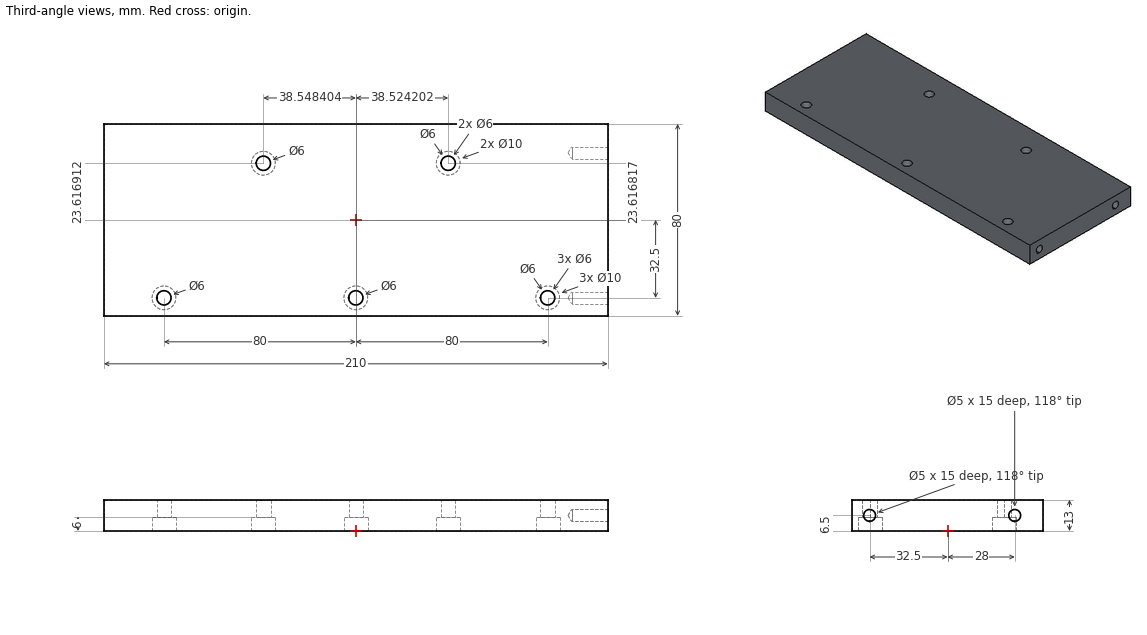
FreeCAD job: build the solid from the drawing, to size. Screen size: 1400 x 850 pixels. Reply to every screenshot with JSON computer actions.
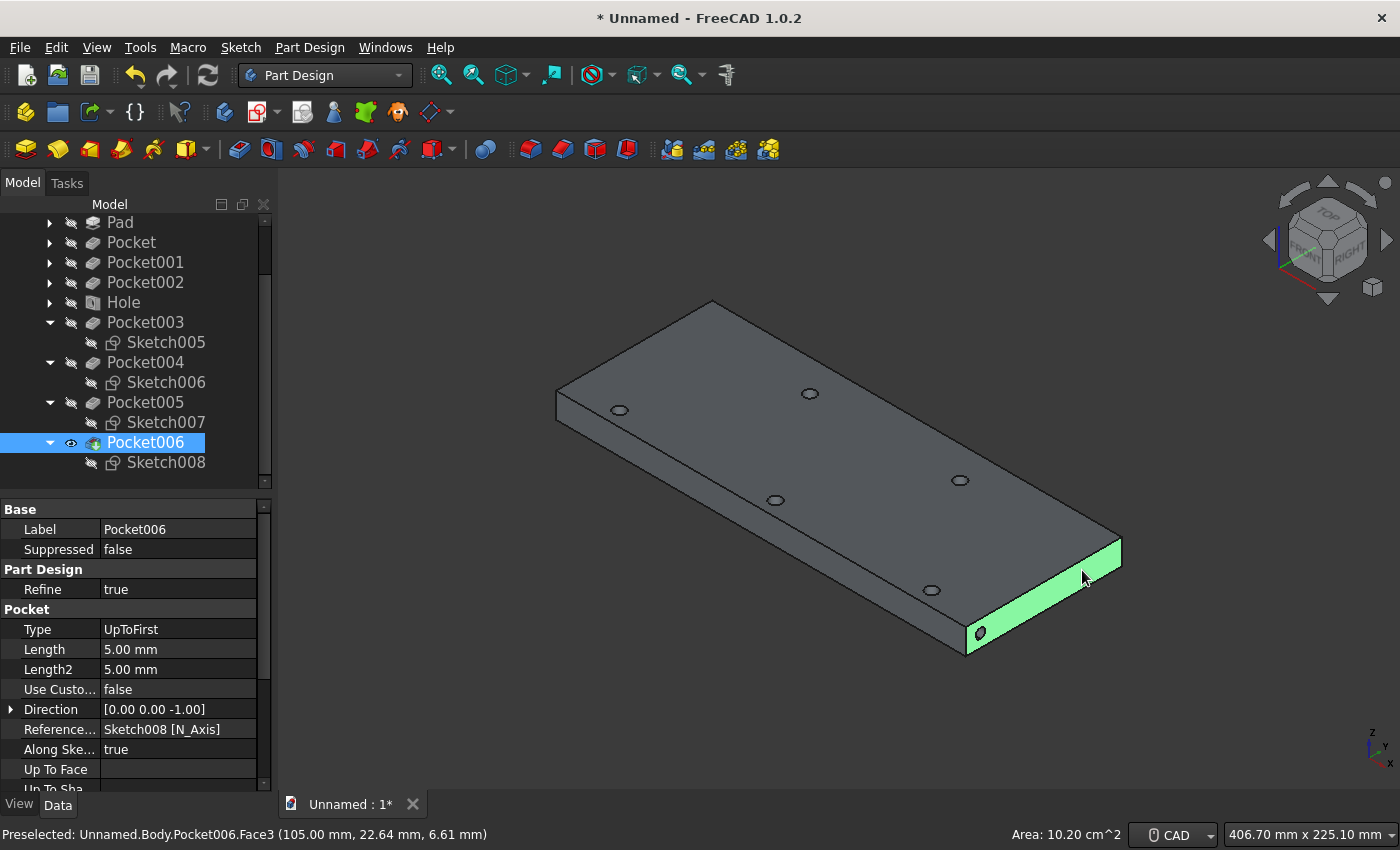
{"action": "left_click", "coordinate": [258, 112]}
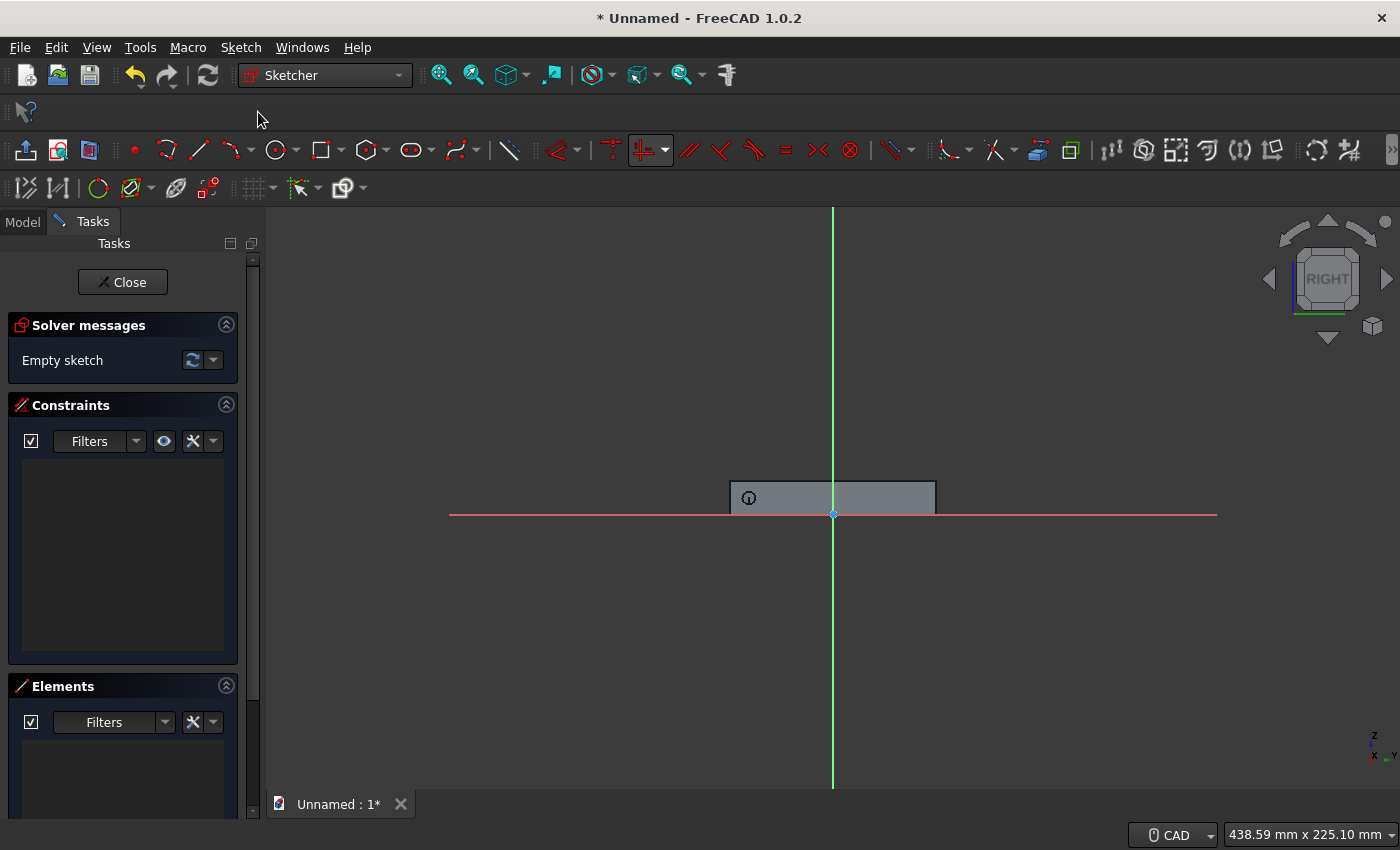
{"action": "scroll", "coordinate": [913, 498], "scroll_direction": "up", "scroll_amount": 15}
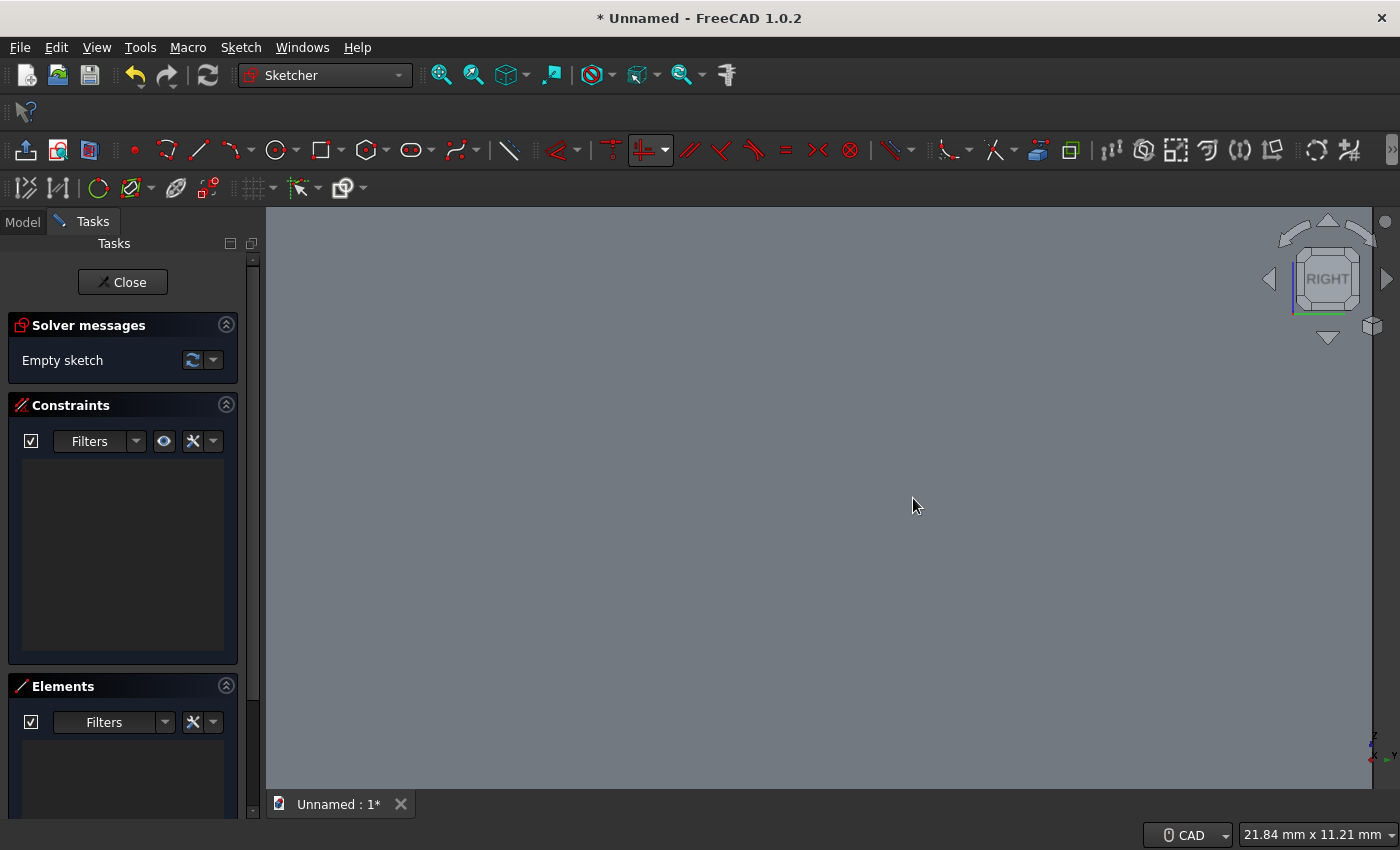
{"action": "scroll", "coordinate": [719, 469], "scroll_direction": "up", "scroll_amount": 2}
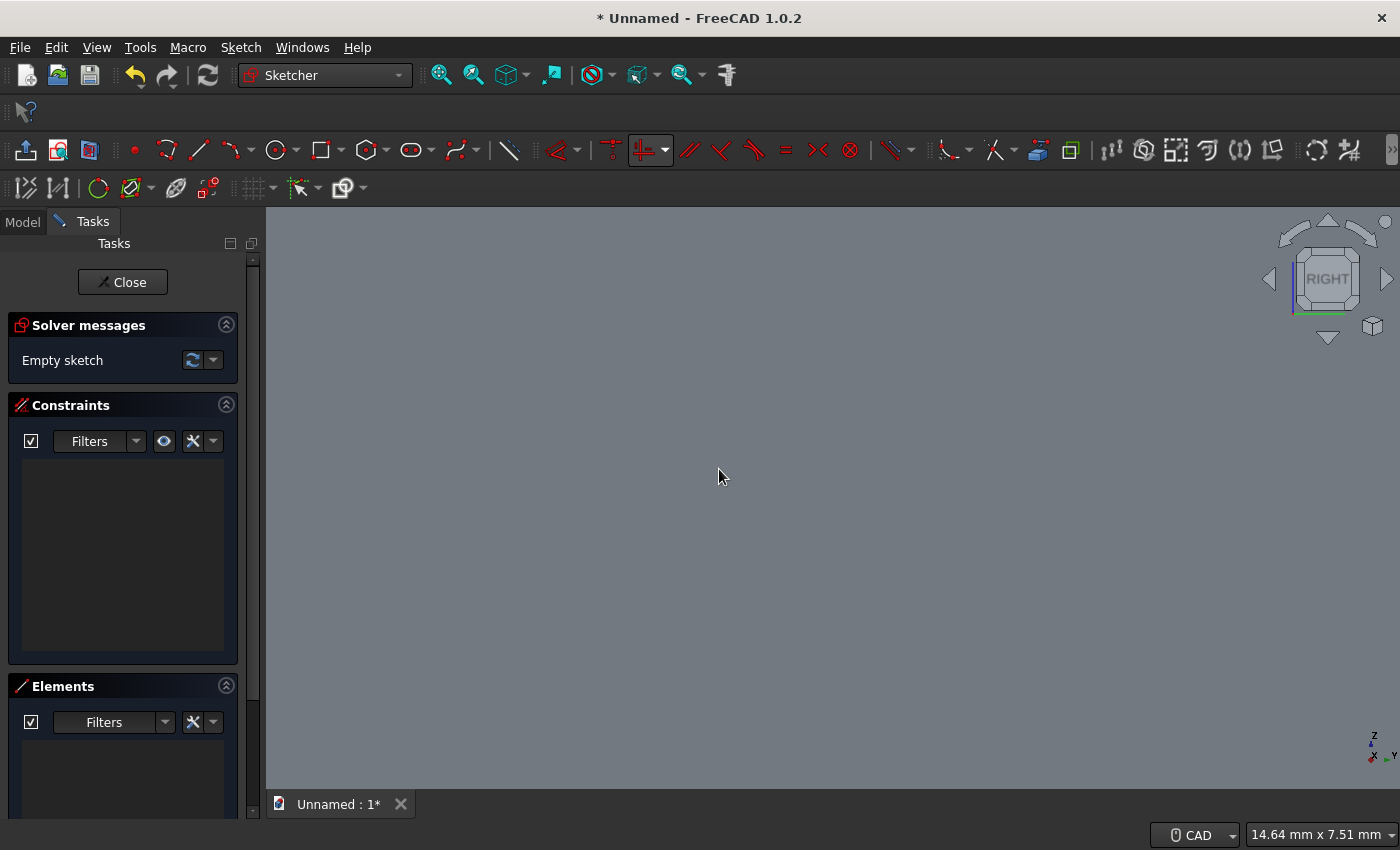
{"action": "key", "text": "g c"}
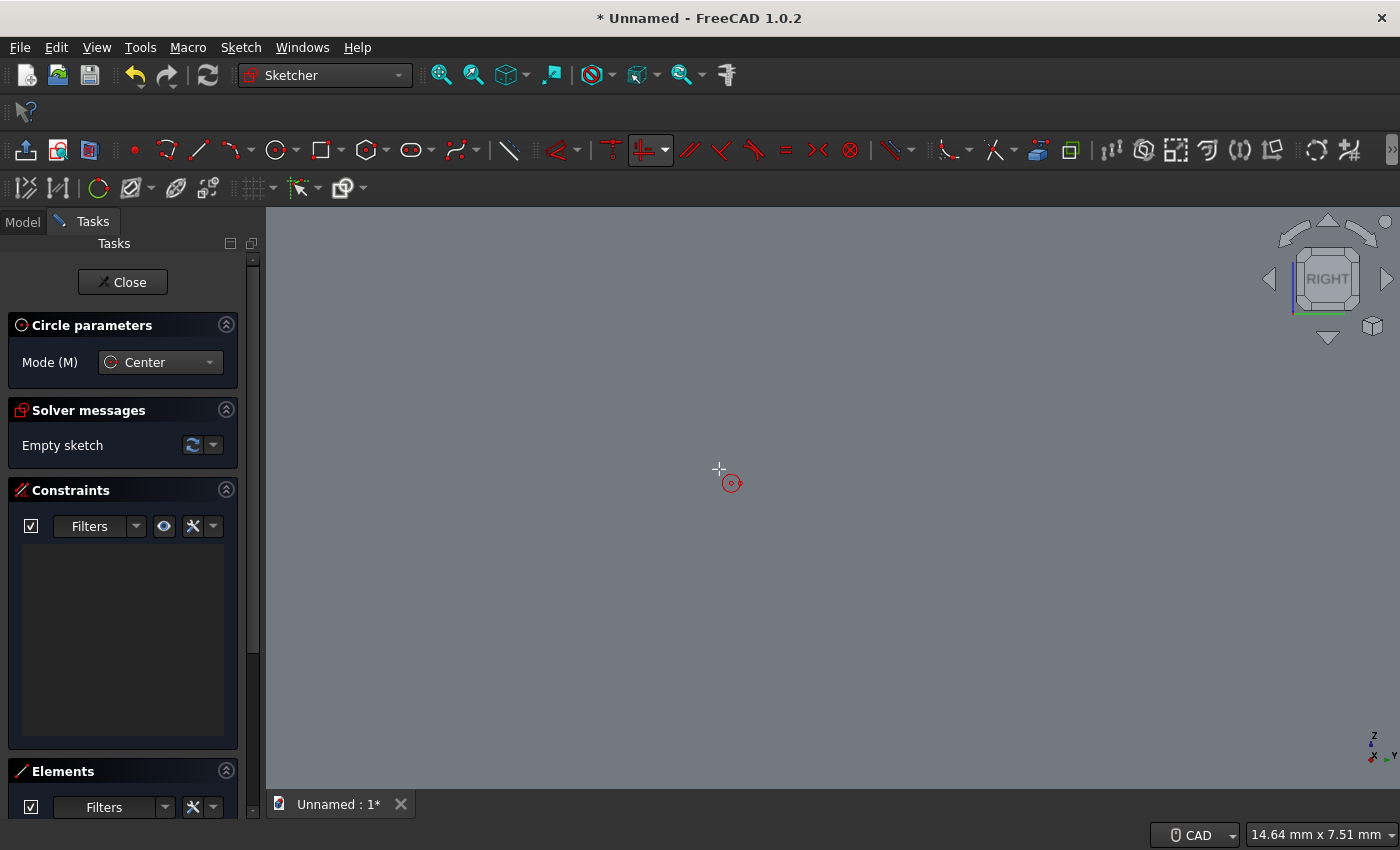
{"action": "left_click", "coordinate": [764, 498]}
{"action": "left_click", "coordinate": [901, 361]}
{"action": "key", "text": "Escape"}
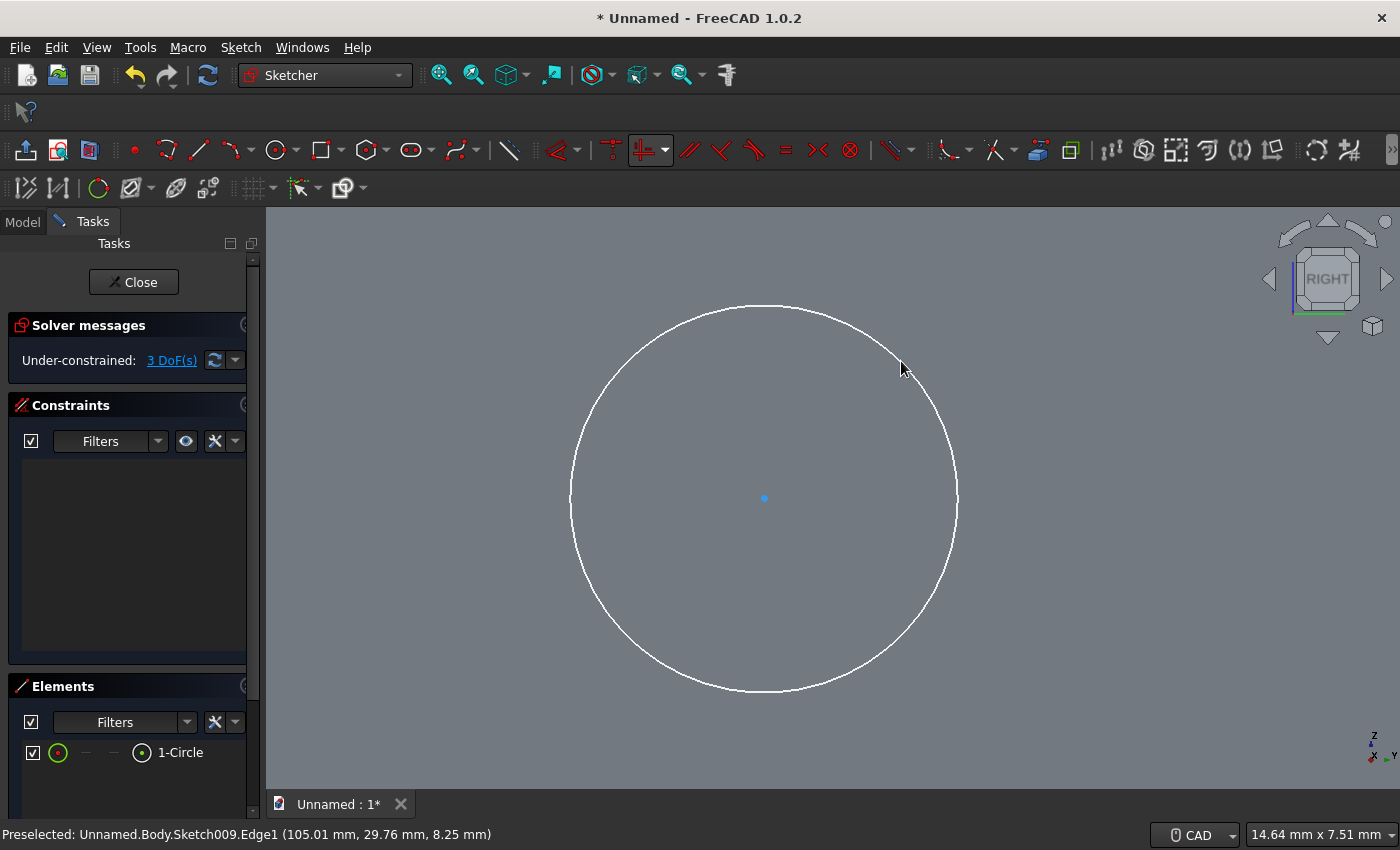
{"action": "left_click", "coordinate": [556, 150]}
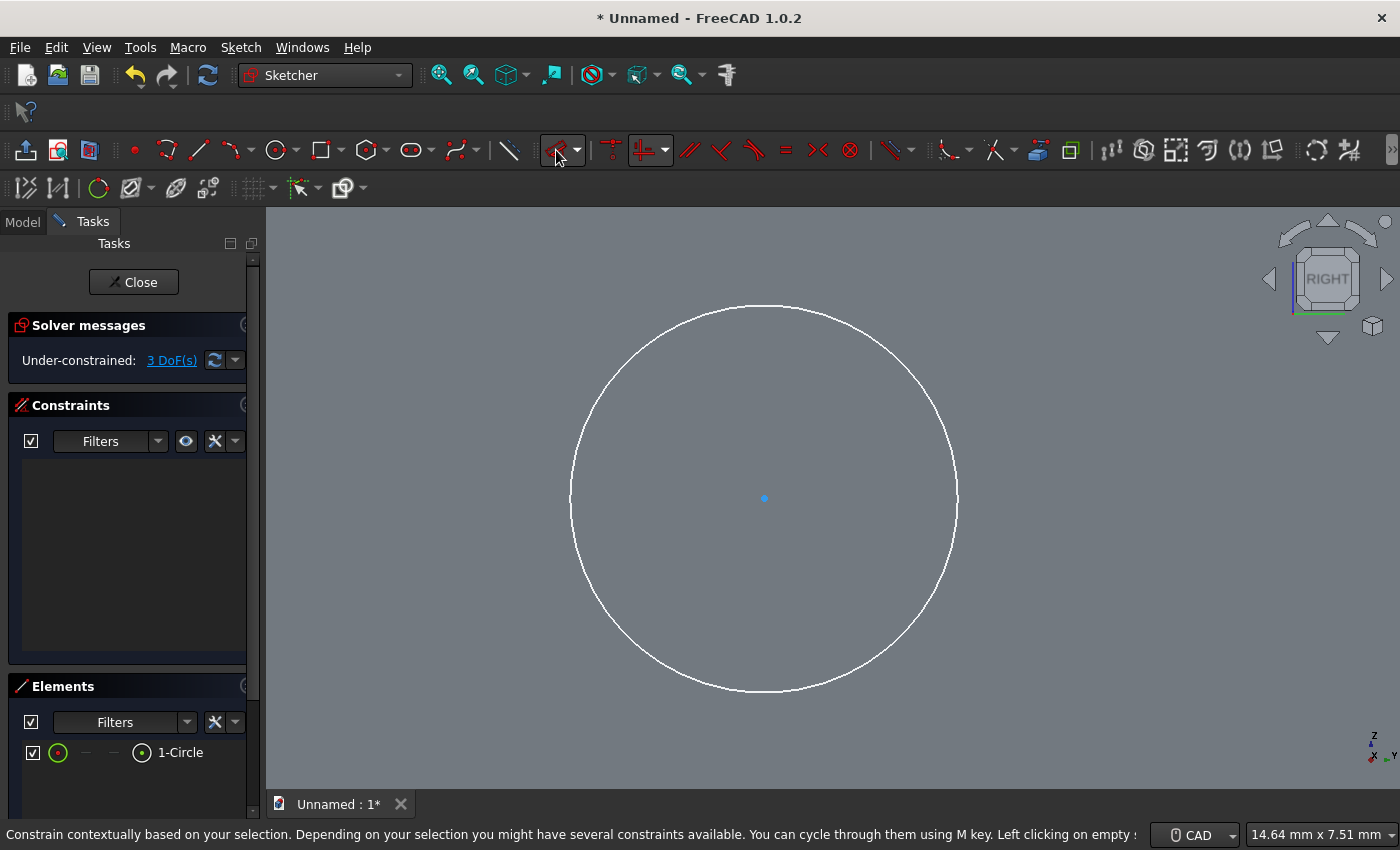
{"action": "left_click", "coordinate": [901, 362]}
{"action": "left_click", "coordinate": [924, 339]}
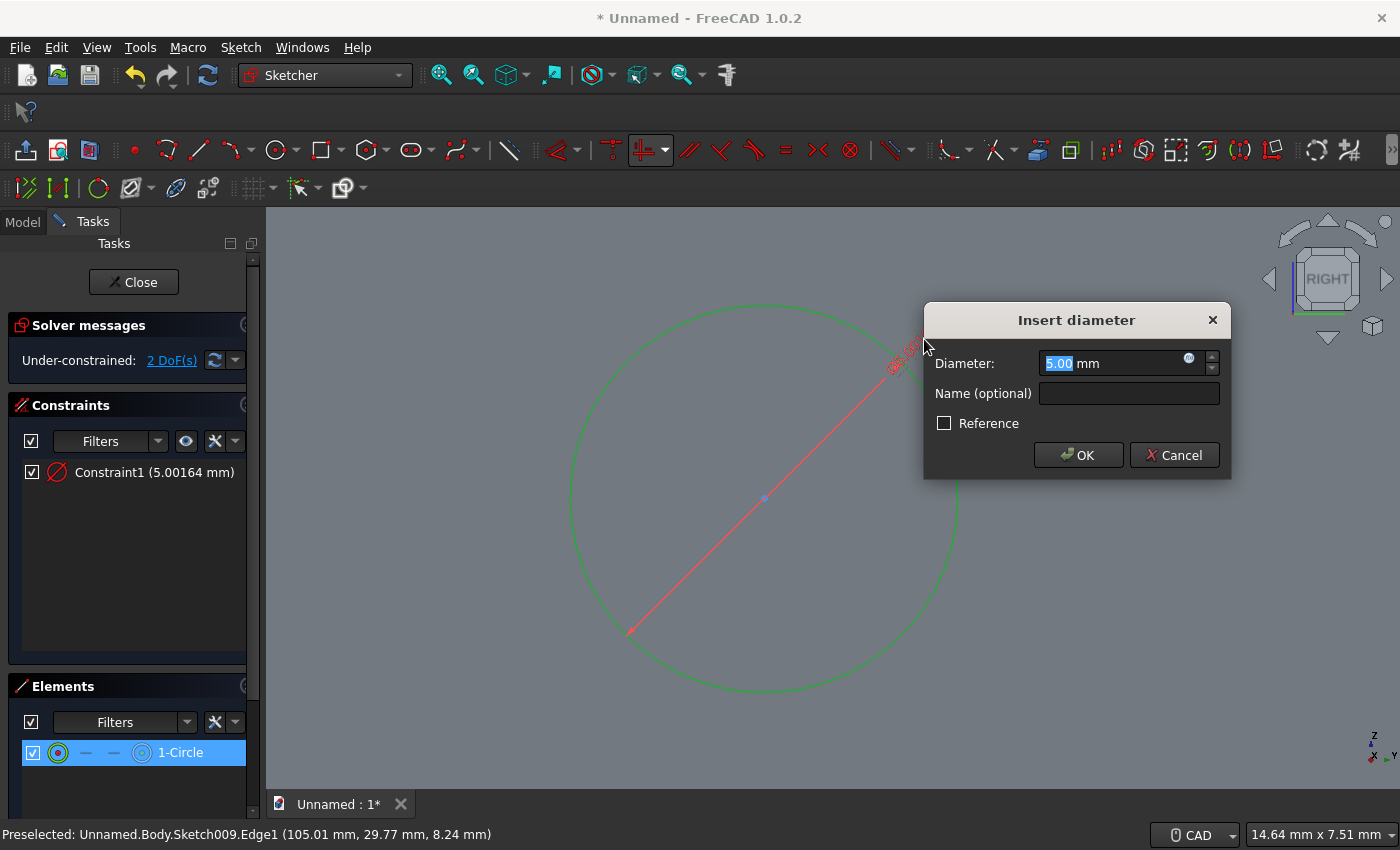
{"action": "type", "text": "5"}
{"action": "key", "text": "Return"}